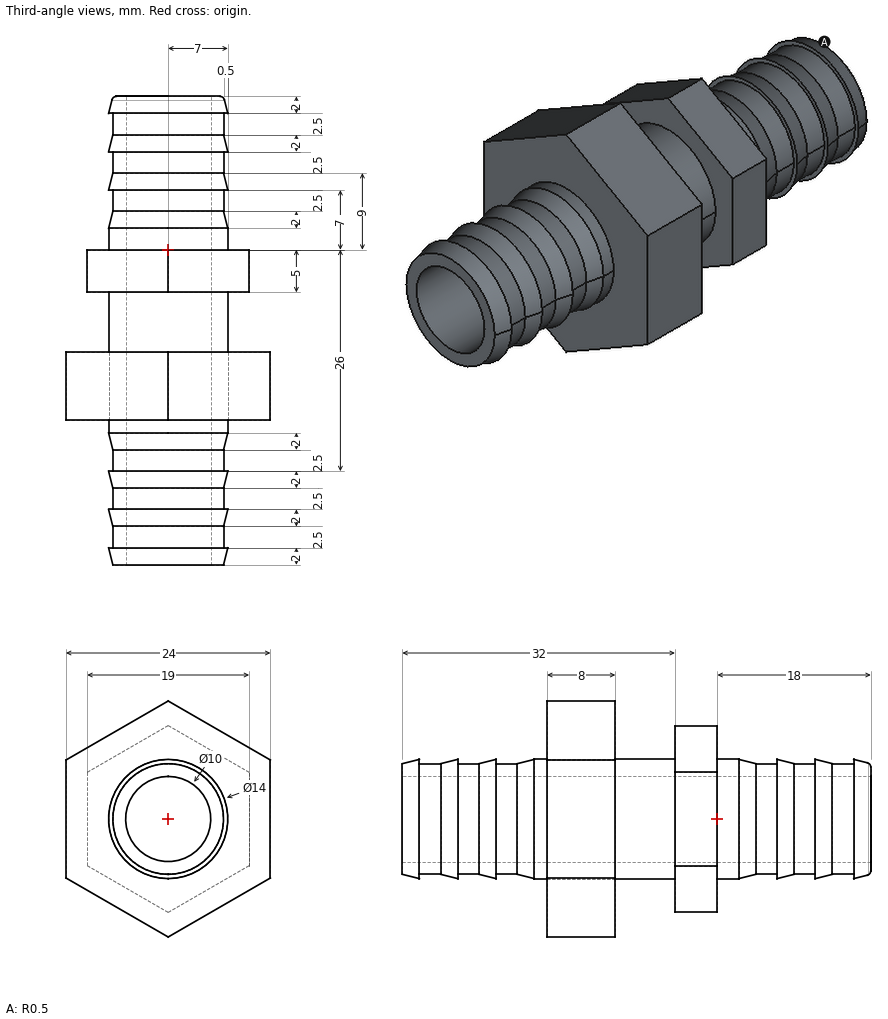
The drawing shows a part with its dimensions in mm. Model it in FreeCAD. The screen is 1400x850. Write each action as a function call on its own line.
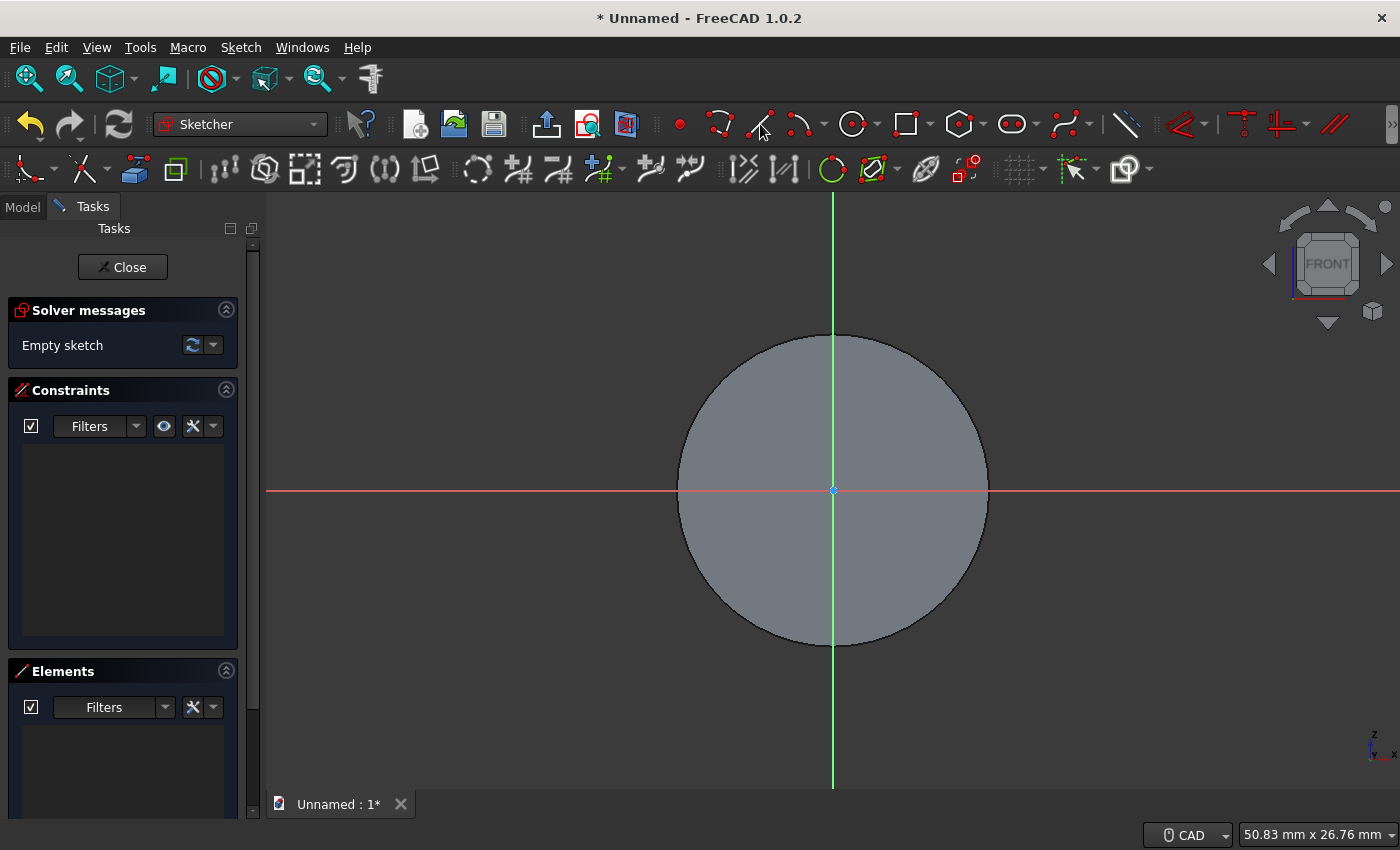
click(960, 124)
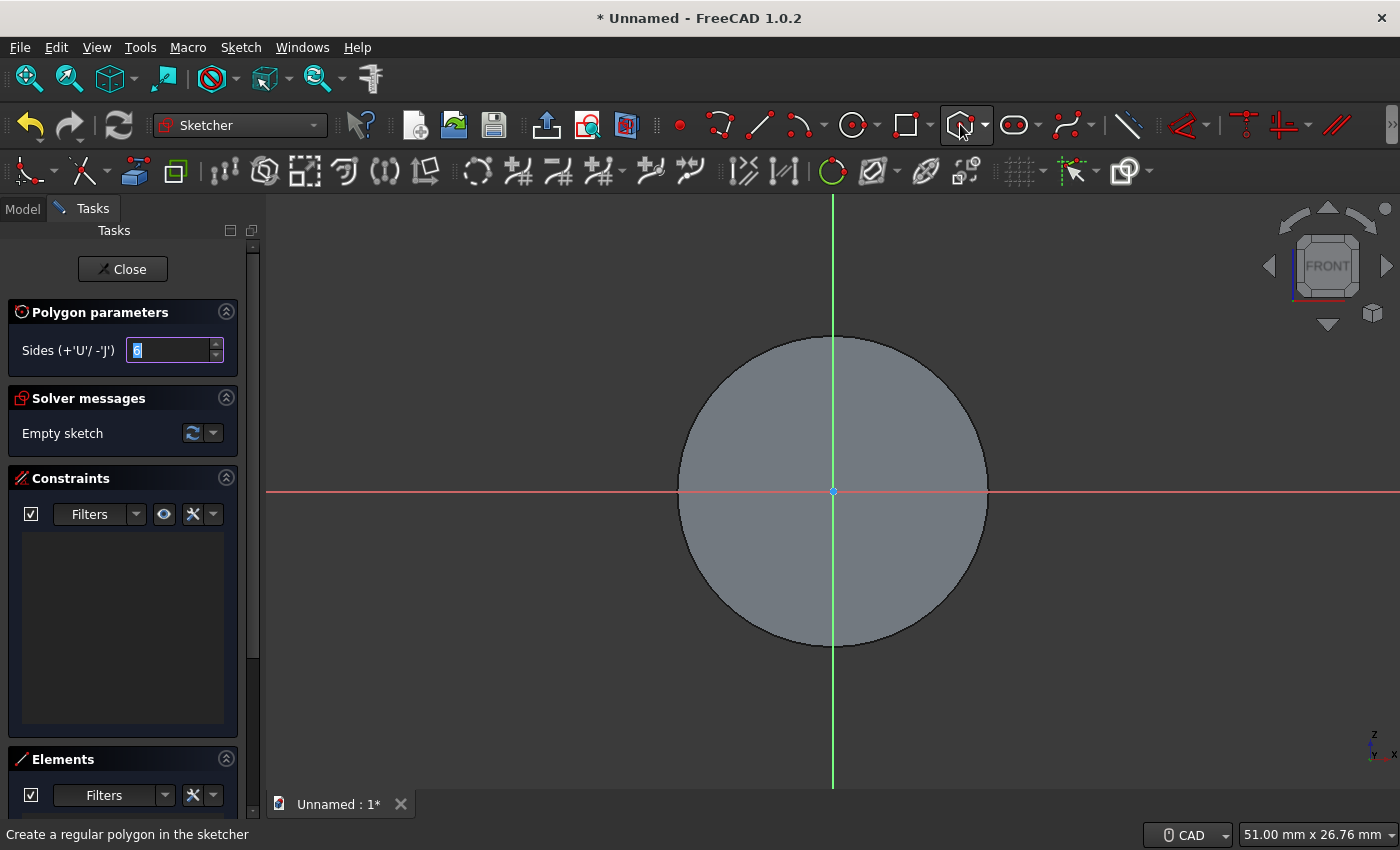
click(833, 492)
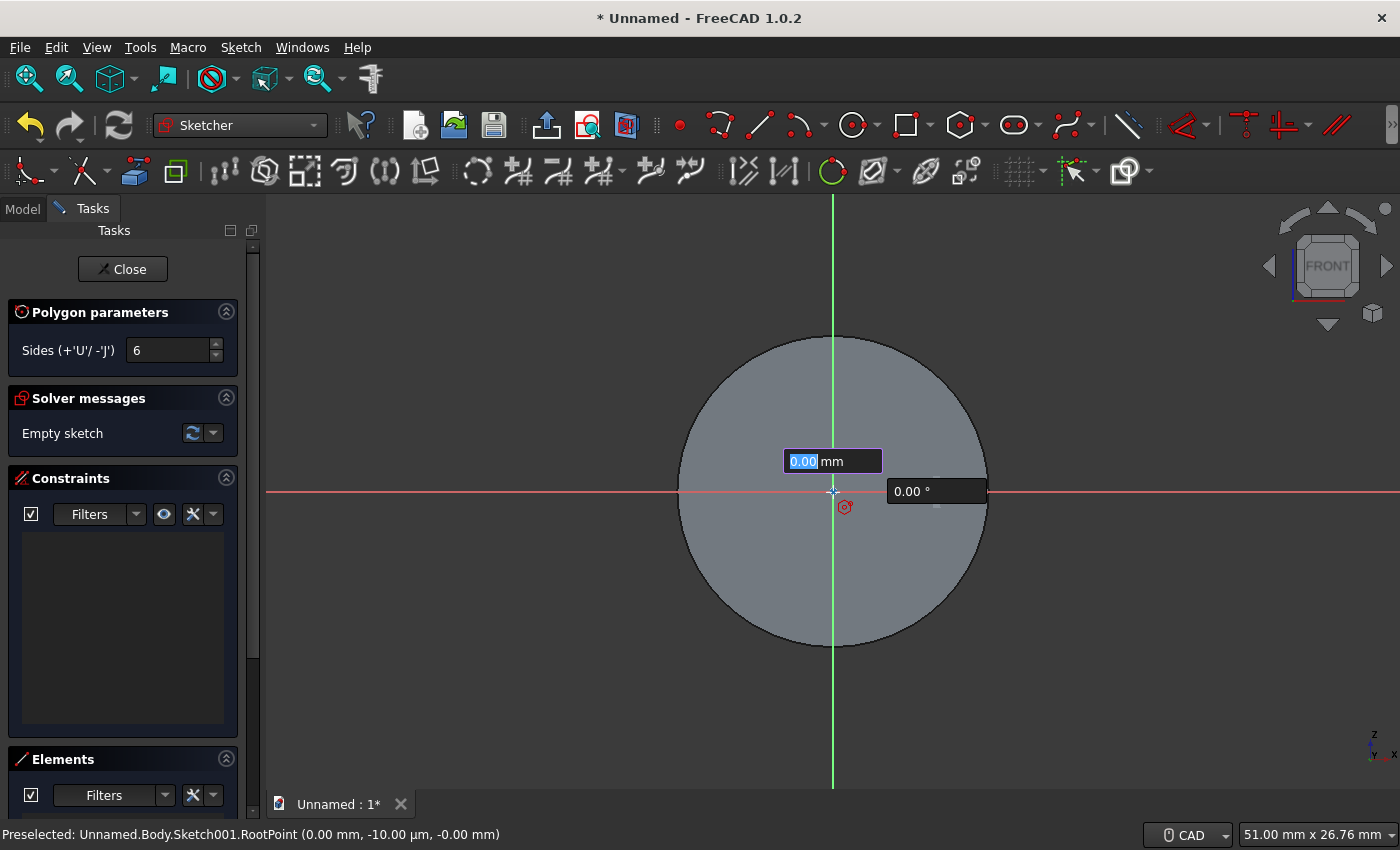
click(833, 248)
right_click(833, 248)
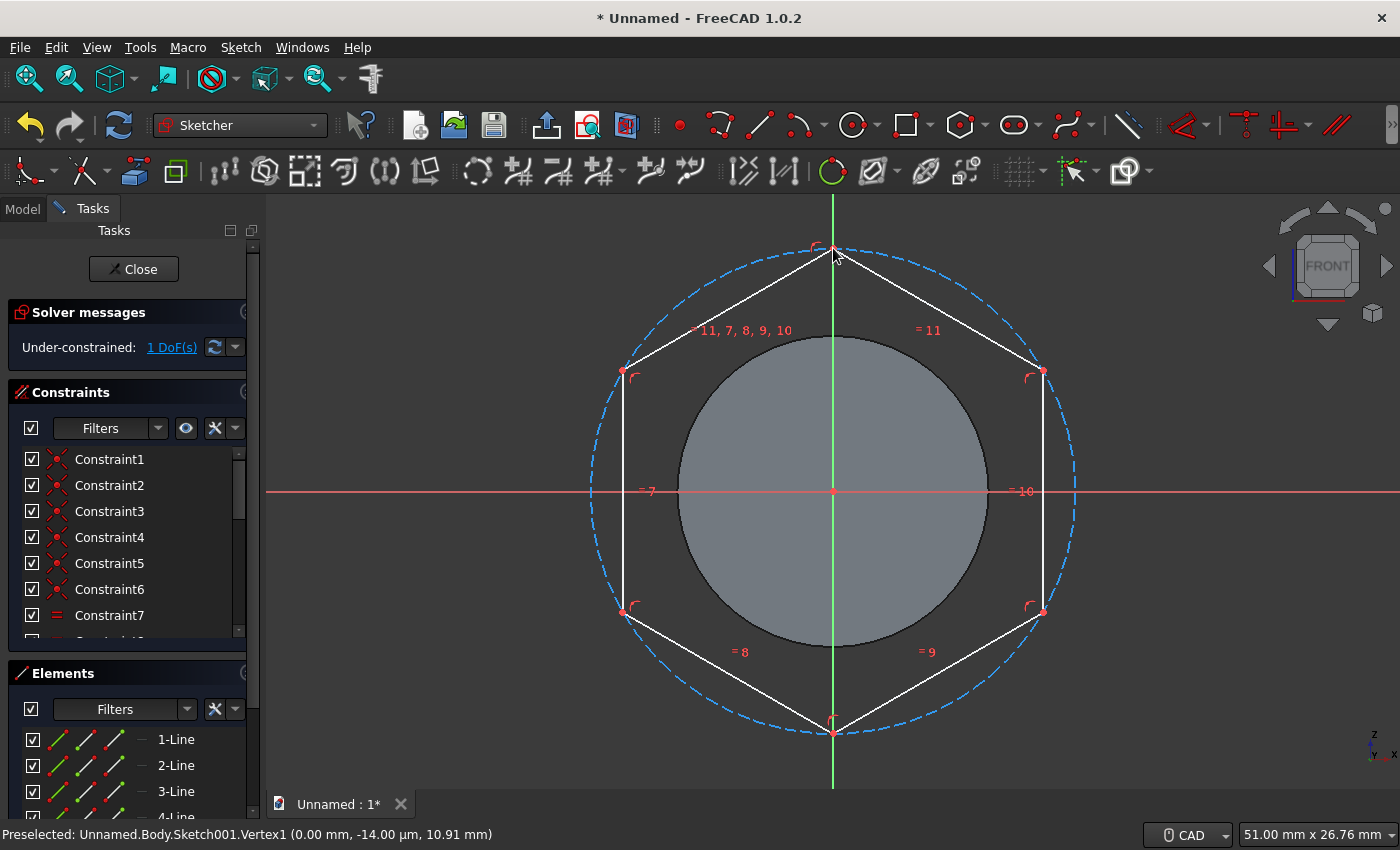
click(1182, 126)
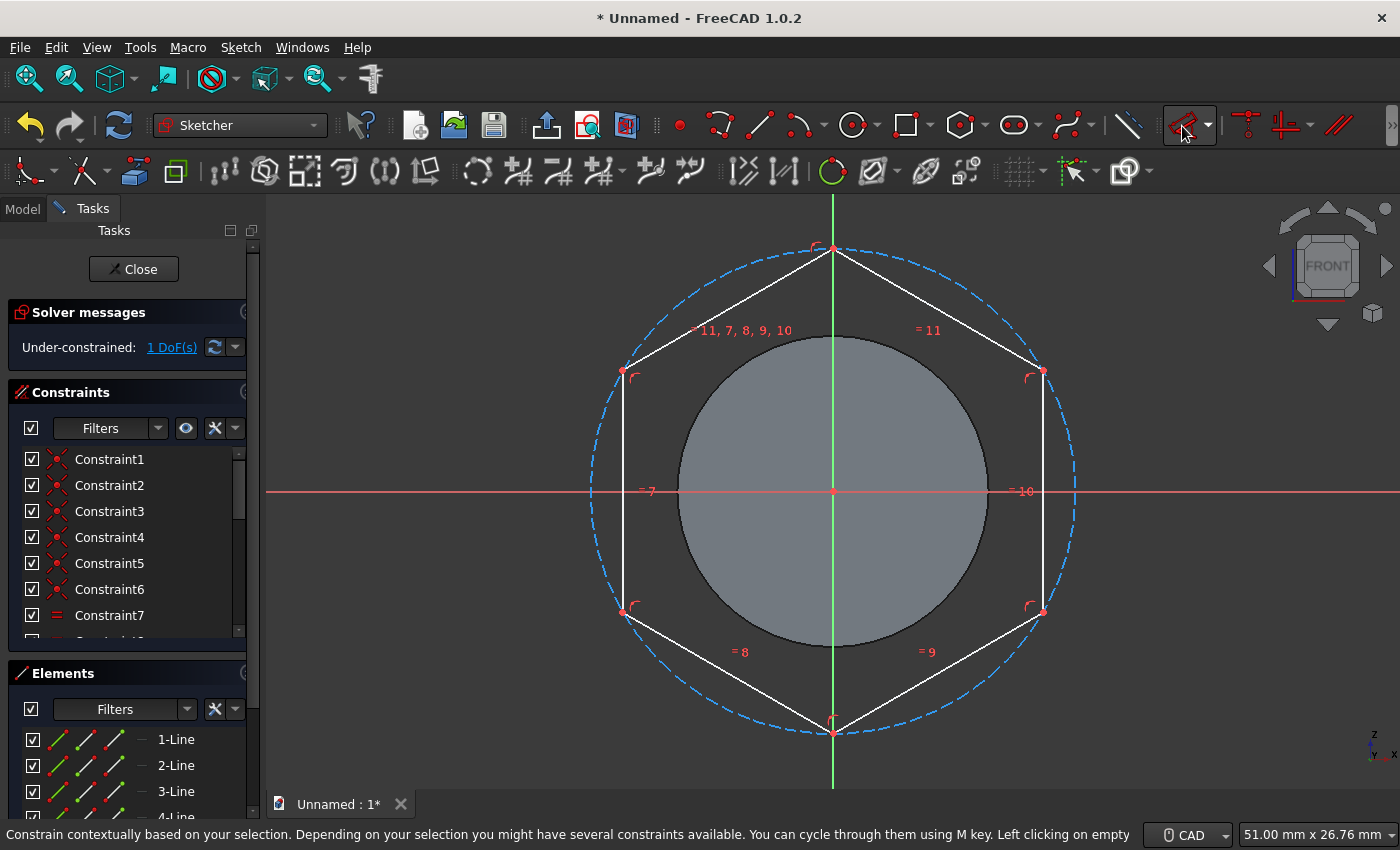
click(623, 370)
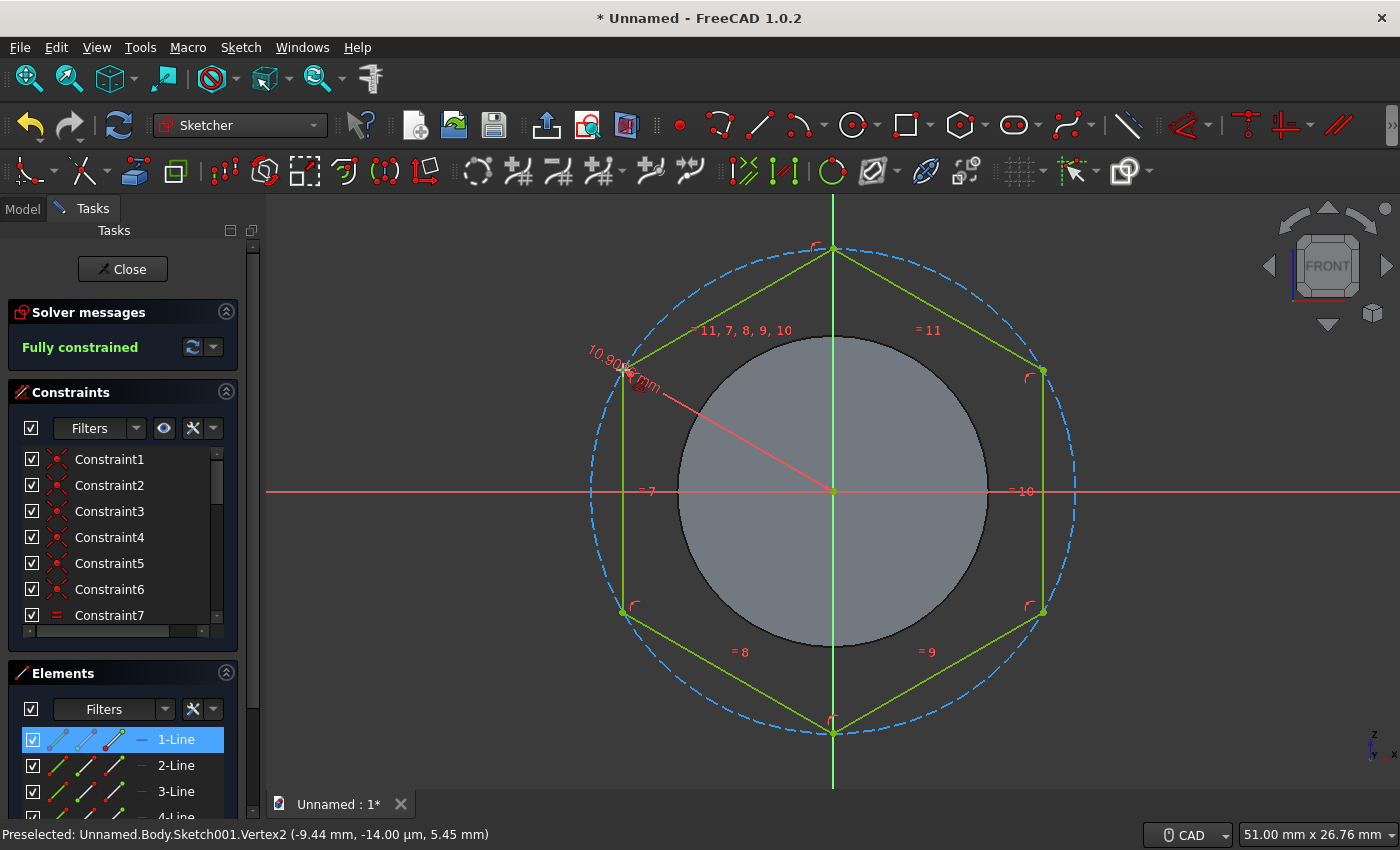
click(1043, 613)
click(736, 647)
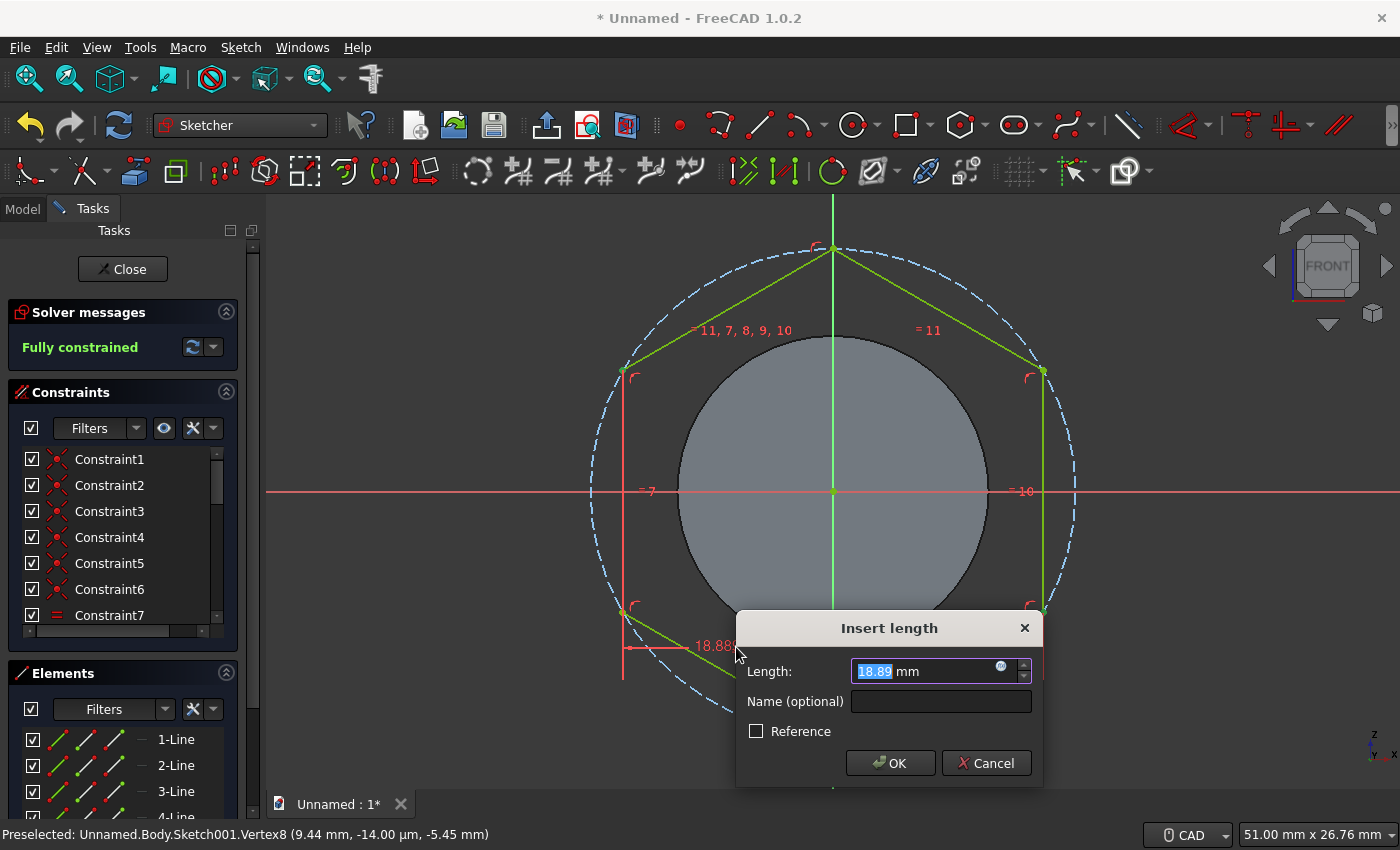
text(19)
key(Return)
key(Escape)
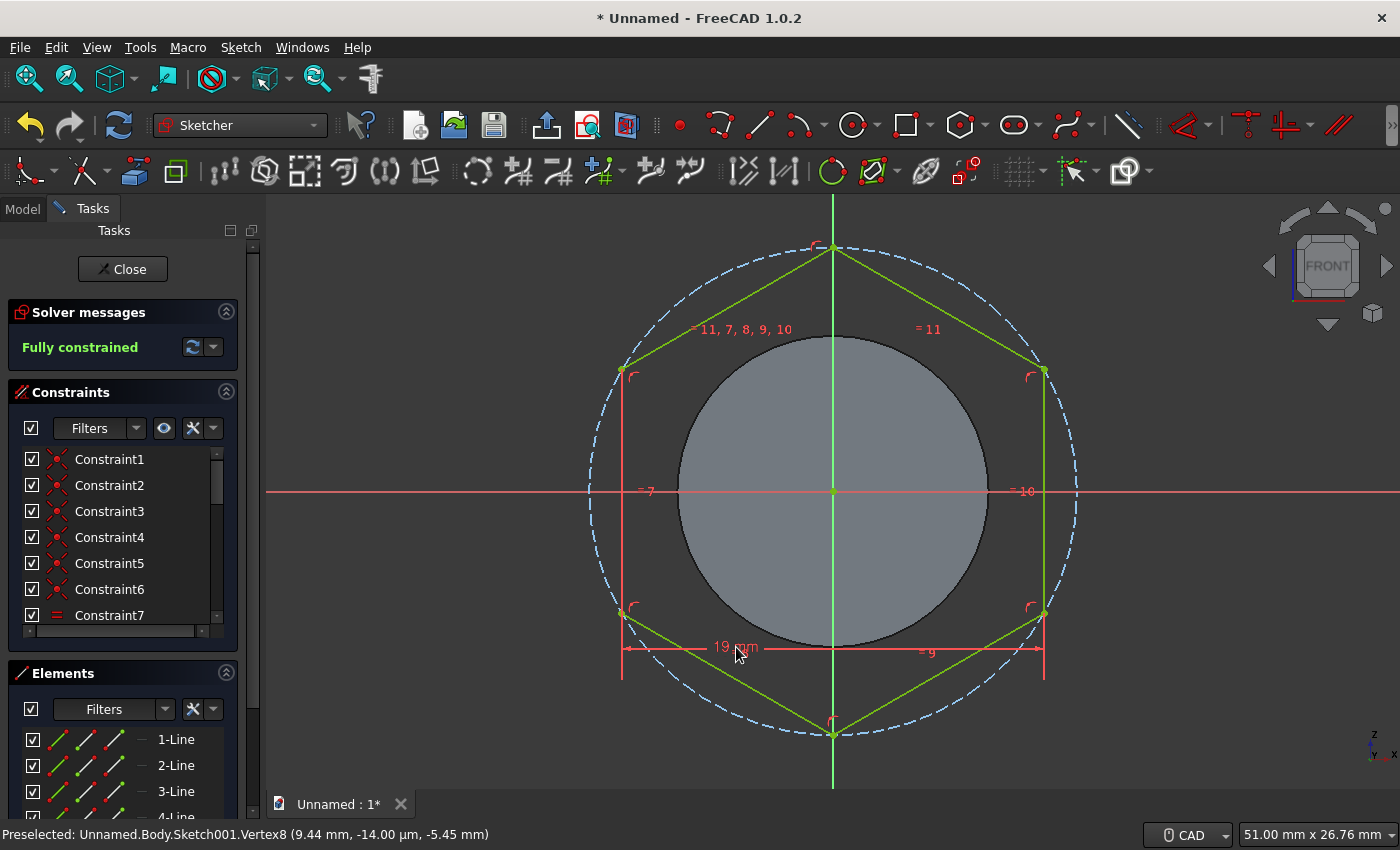
click(123, 269)